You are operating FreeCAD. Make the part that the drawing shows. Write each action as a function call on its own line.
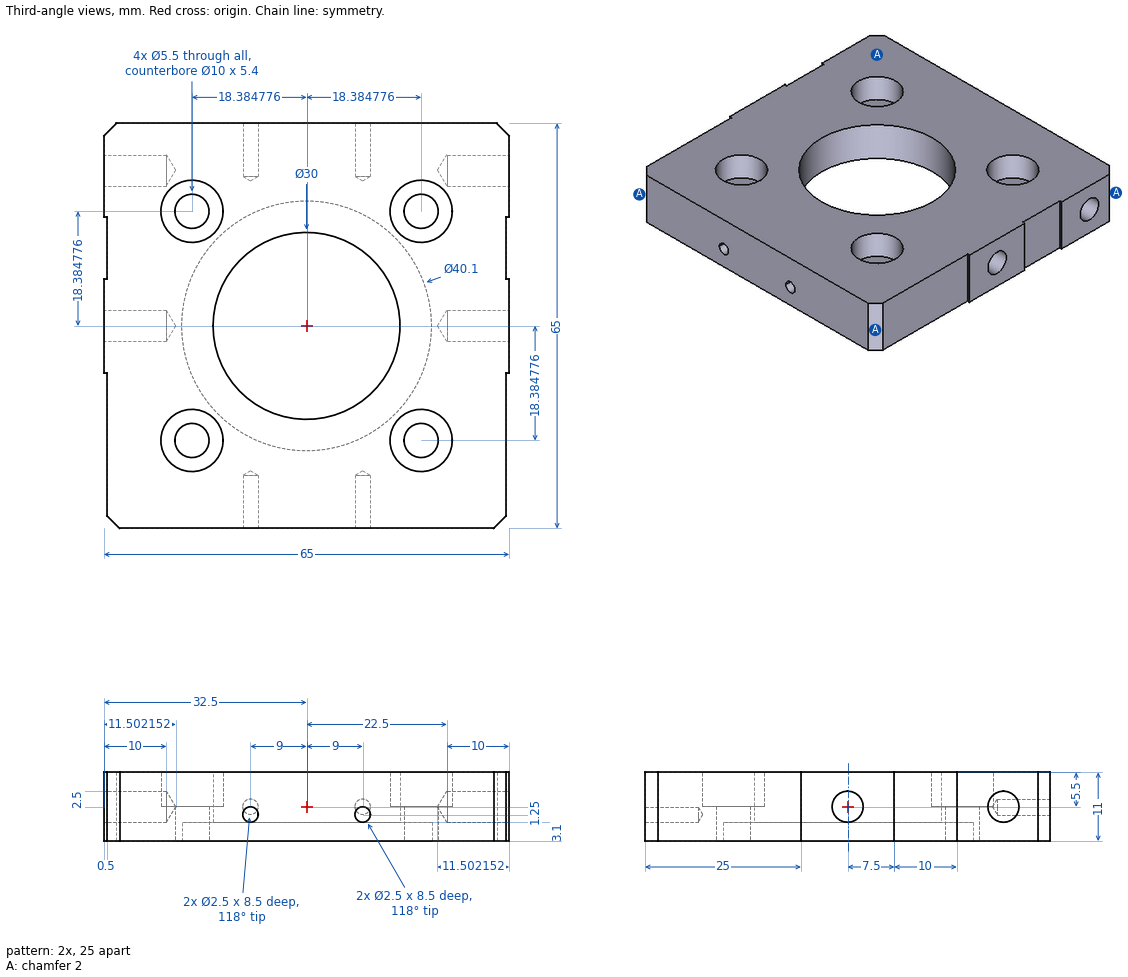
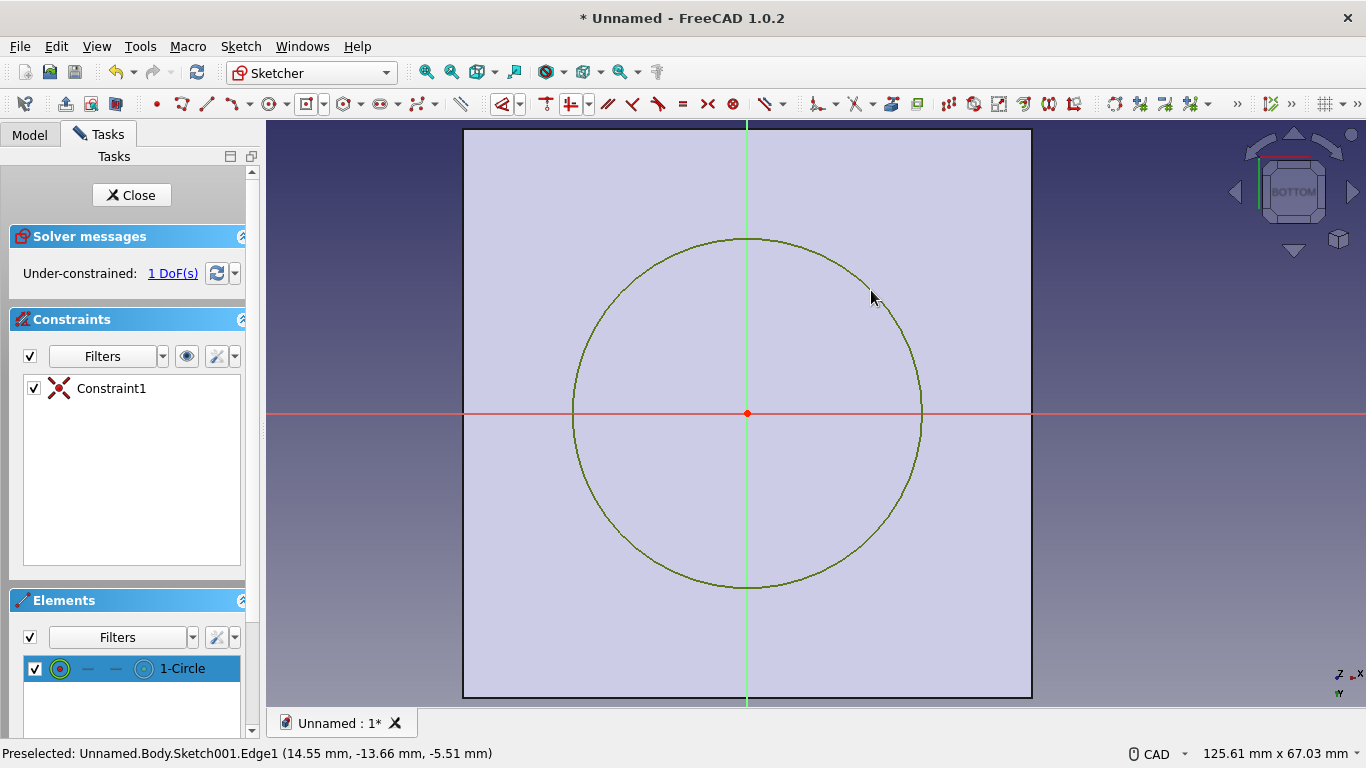
click(520, 104)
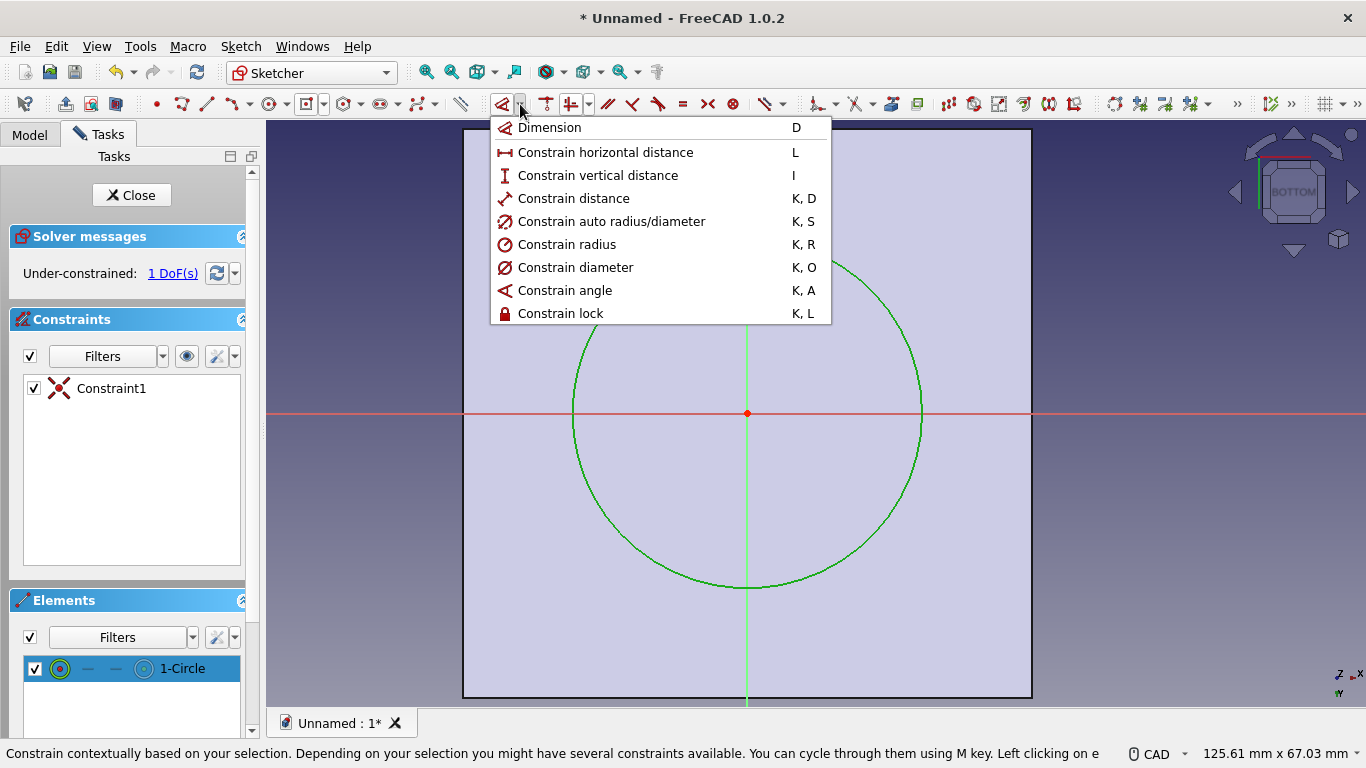
click(661, 268)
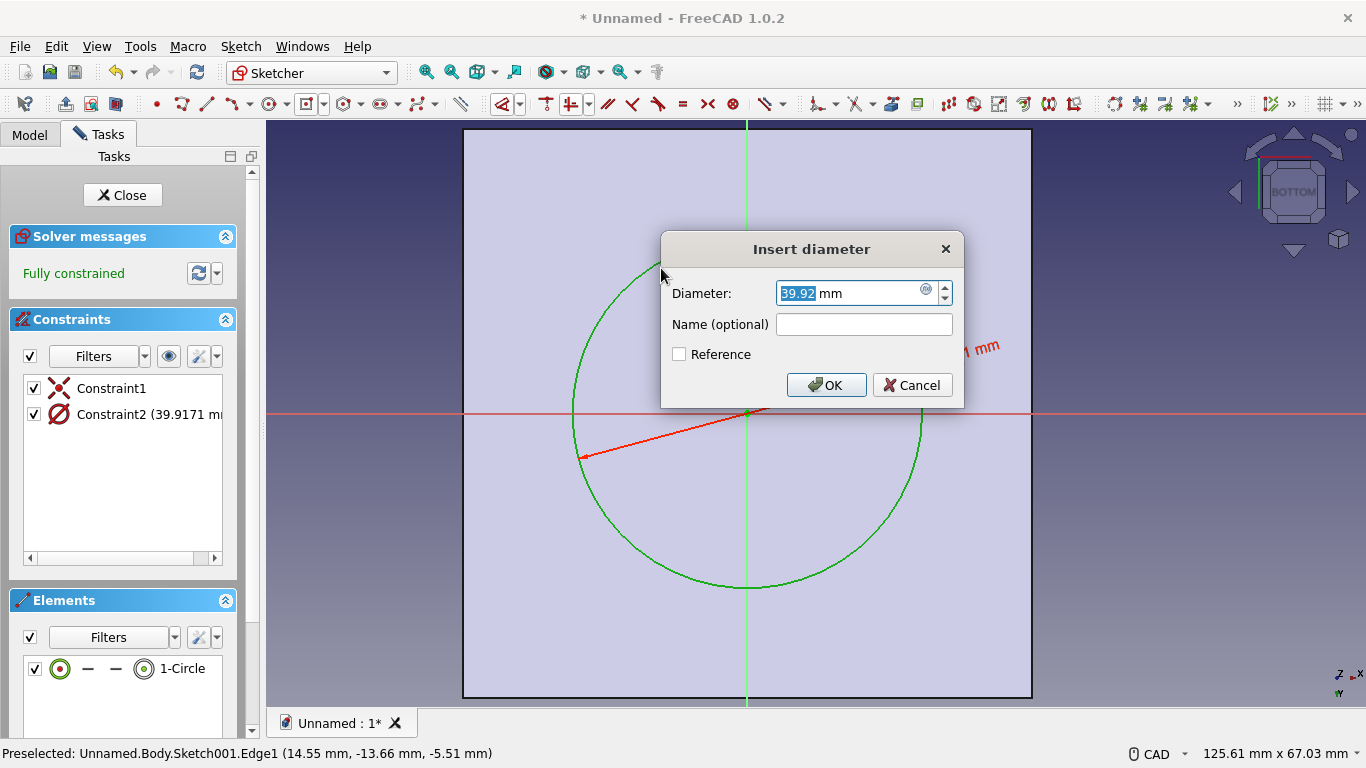
text(40.1)
key(Return)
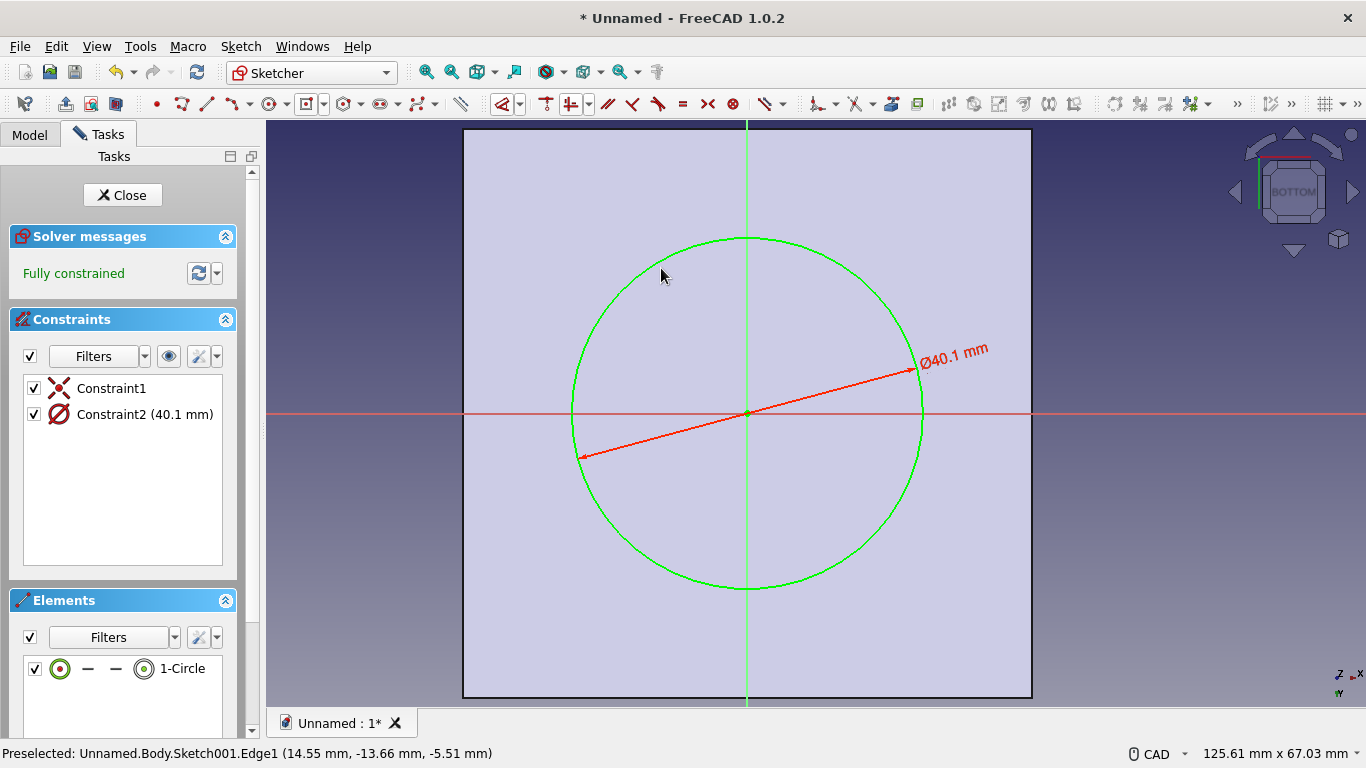
click(123, 195)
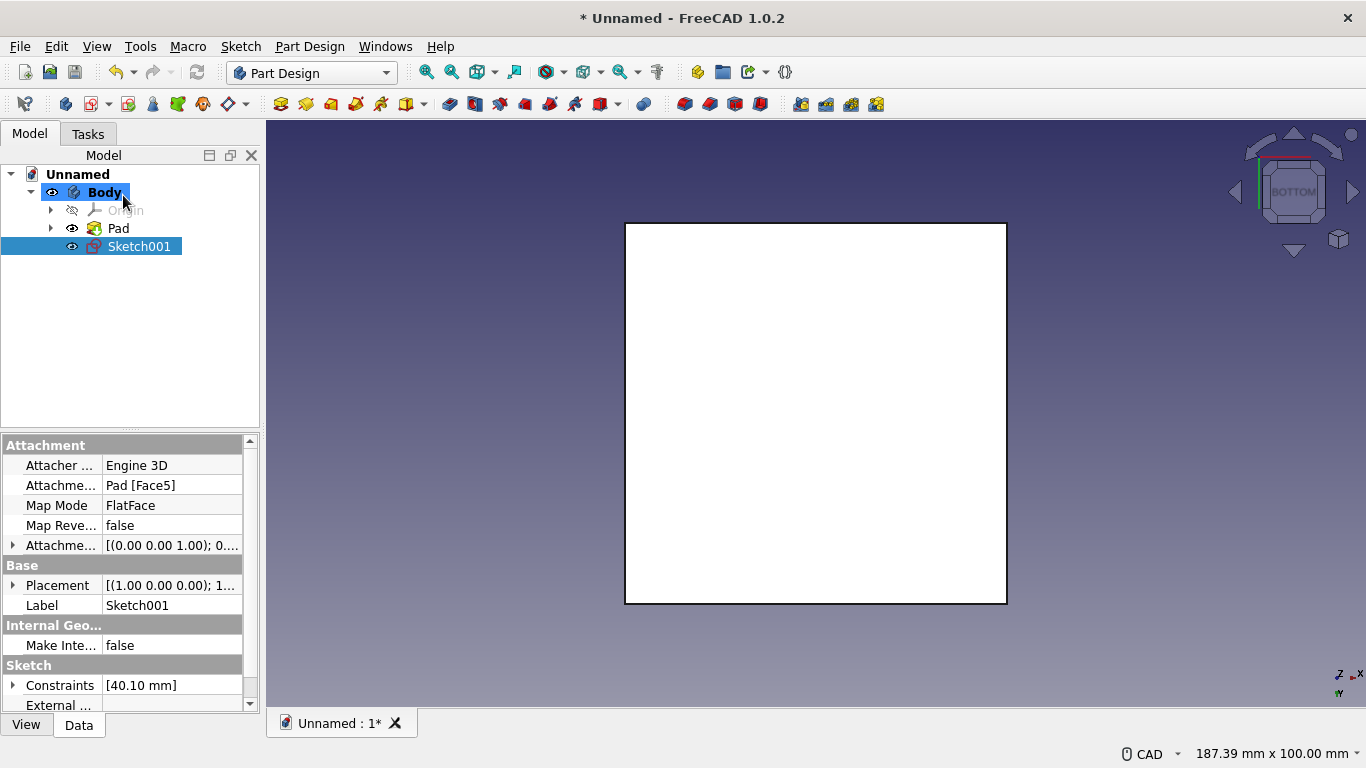
click(450, 104)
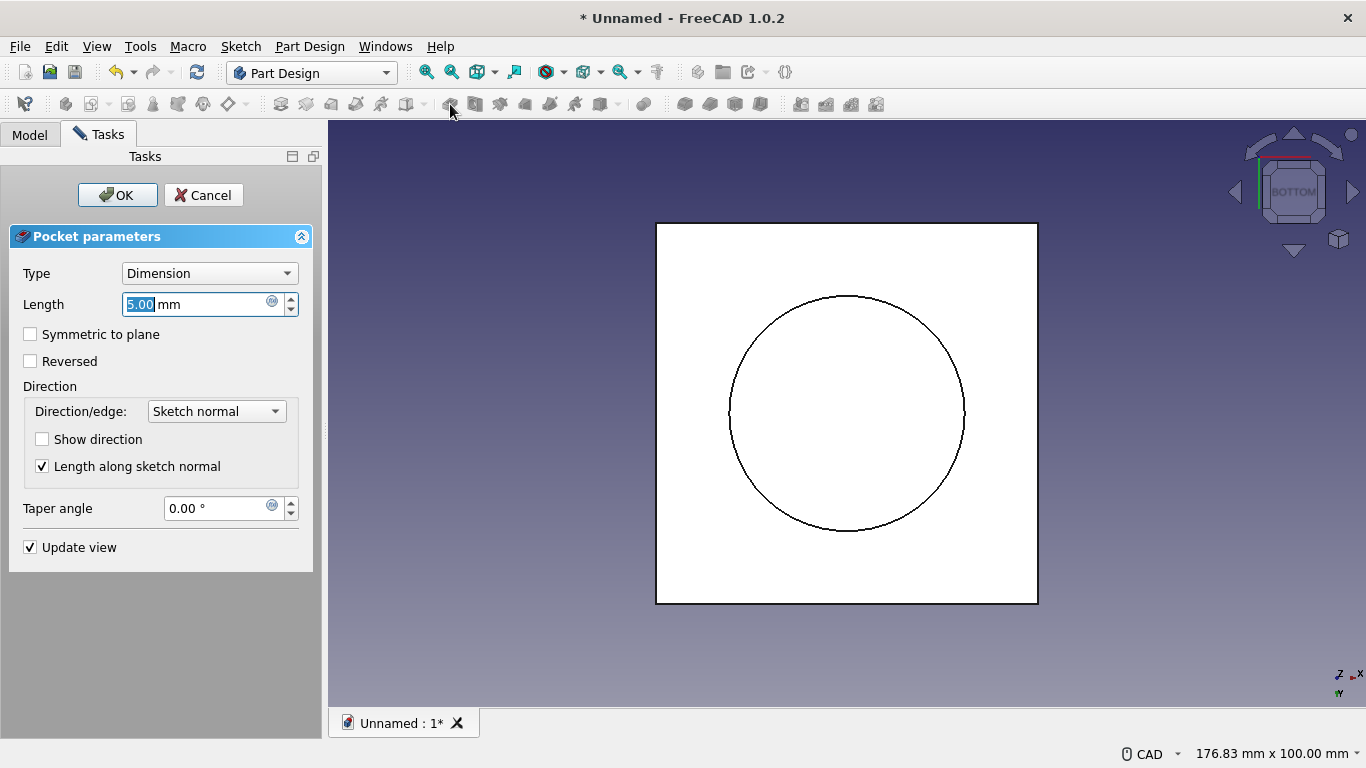
text(3.1)
key(Tab)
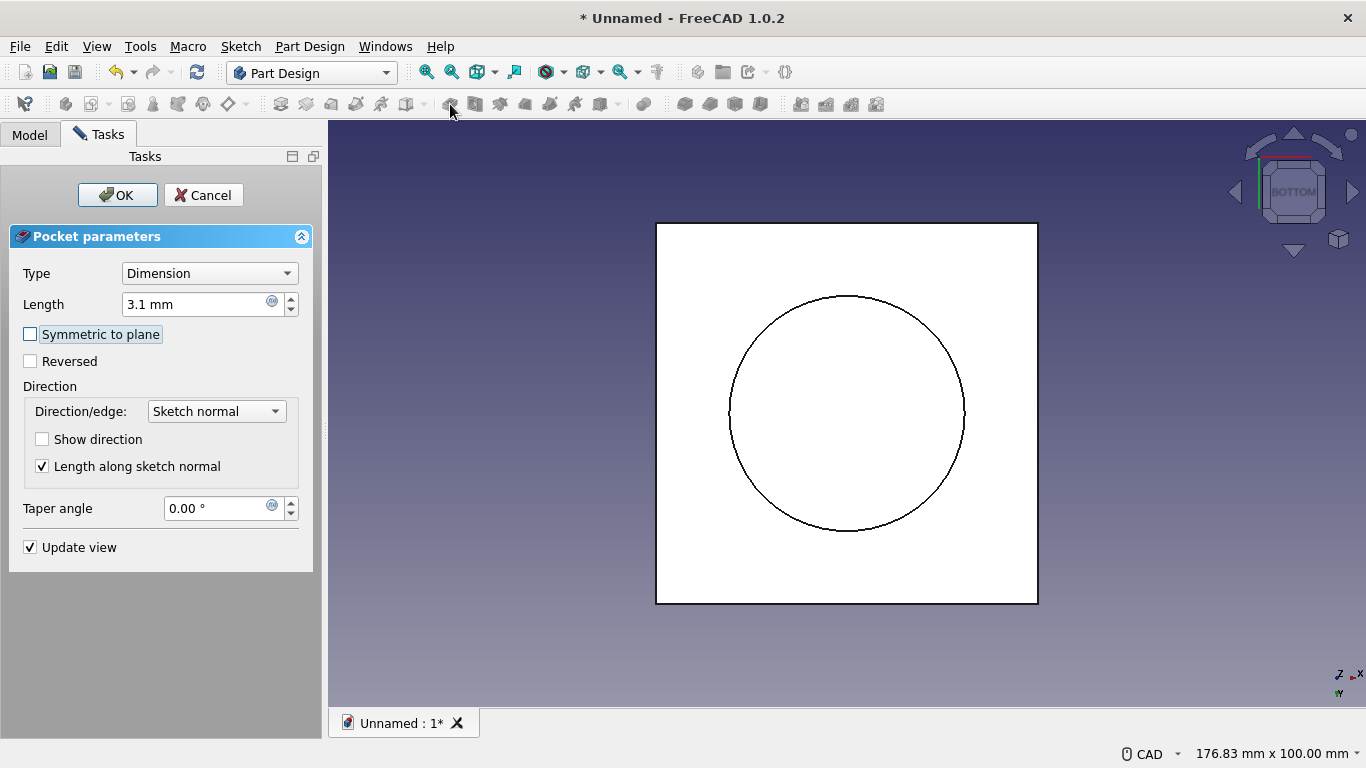
click(118, 195)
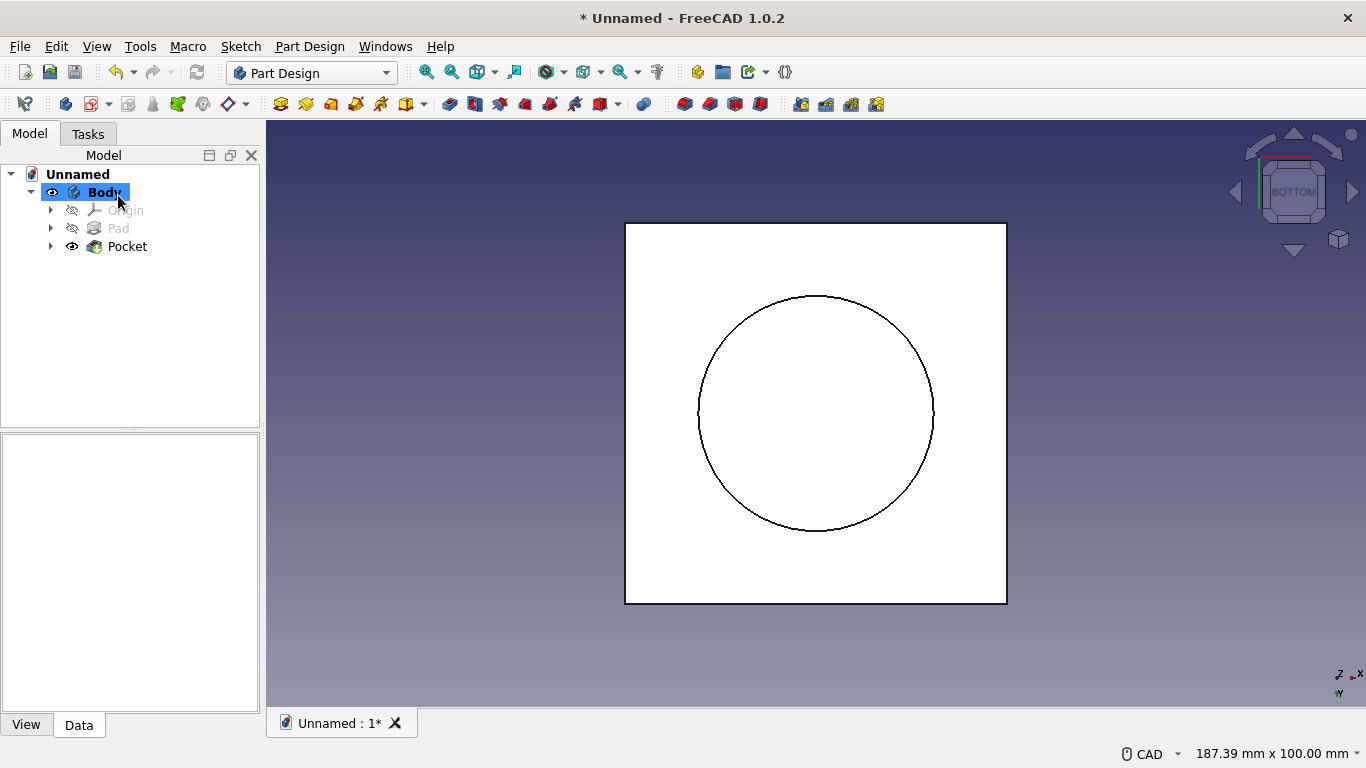
click(816, 413)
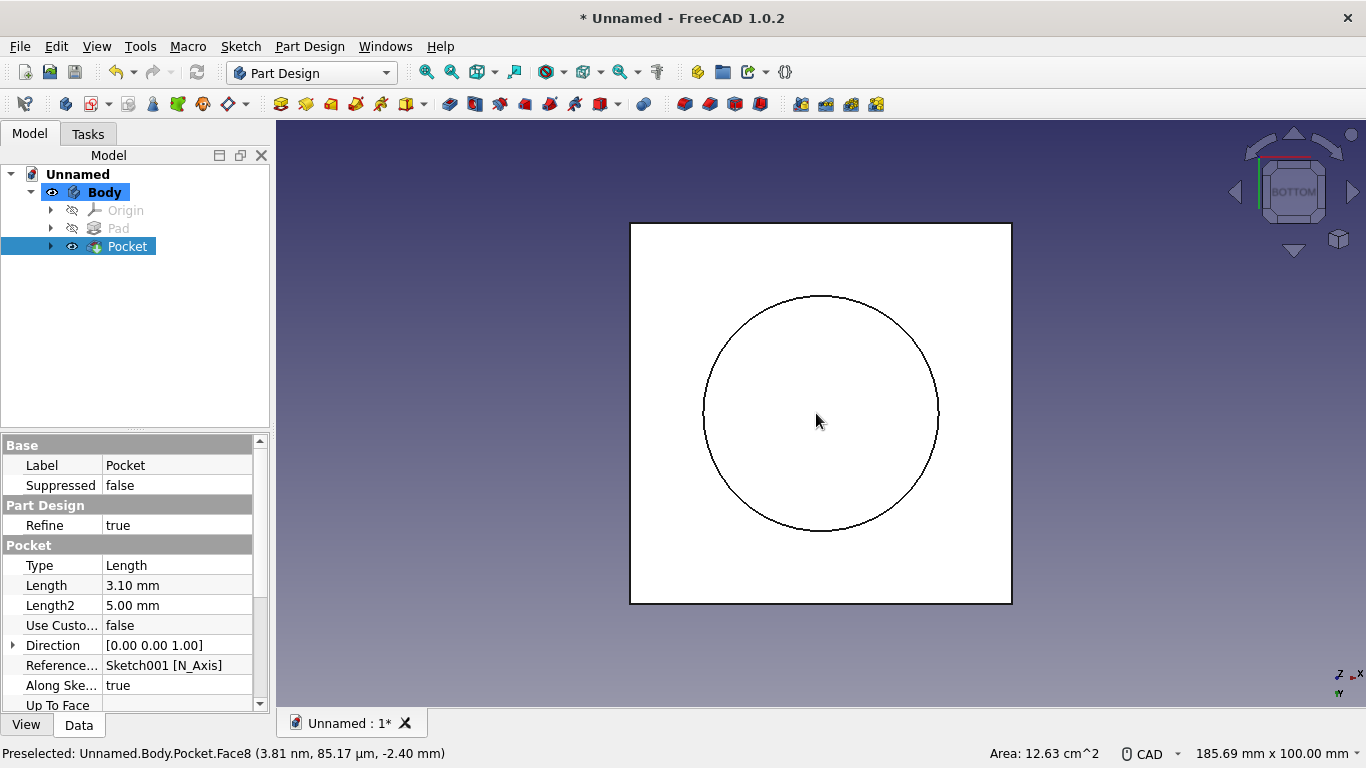
click(90, 104)